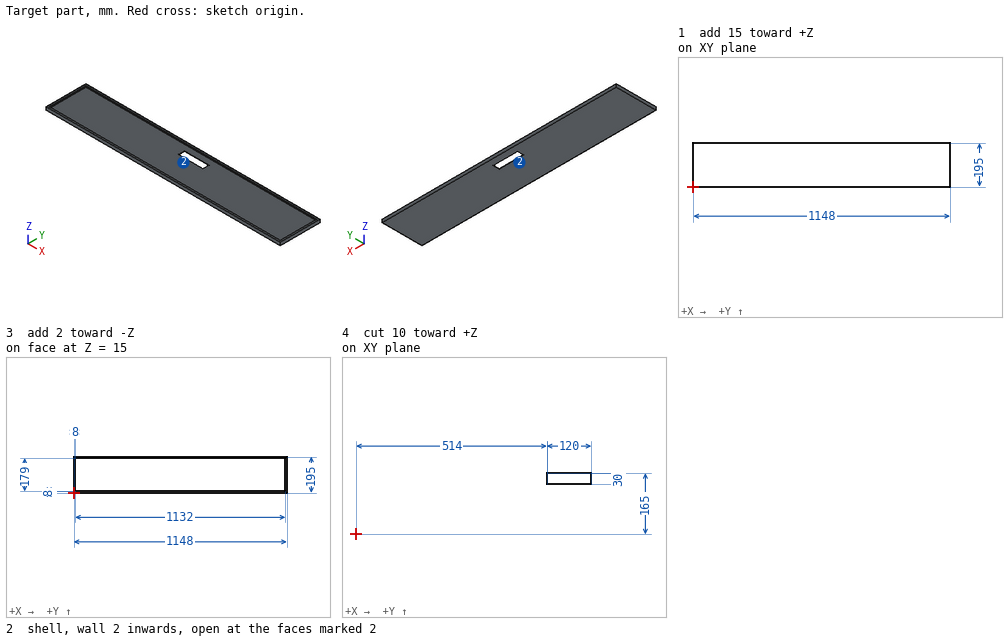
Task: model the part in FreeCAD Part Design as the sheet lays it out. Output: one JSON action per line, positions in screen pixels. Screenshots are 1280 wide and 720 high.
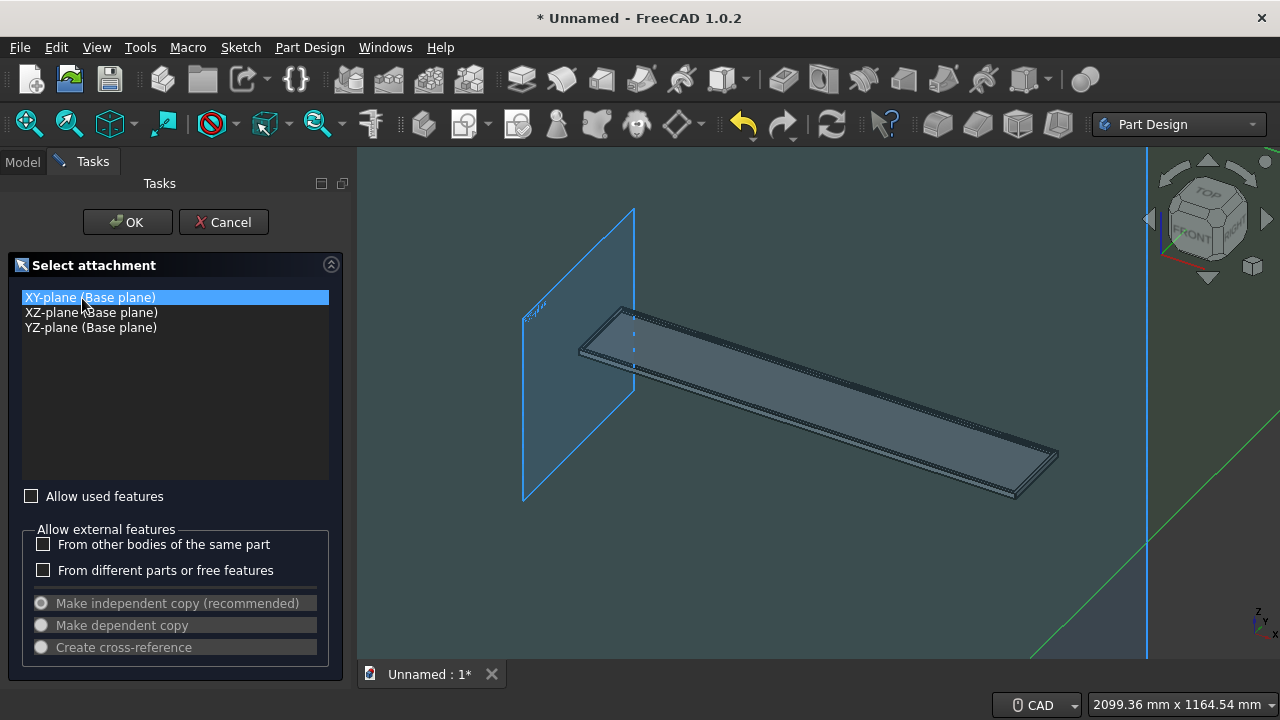
{"action": "left_click", "coordinate": [128, 222]}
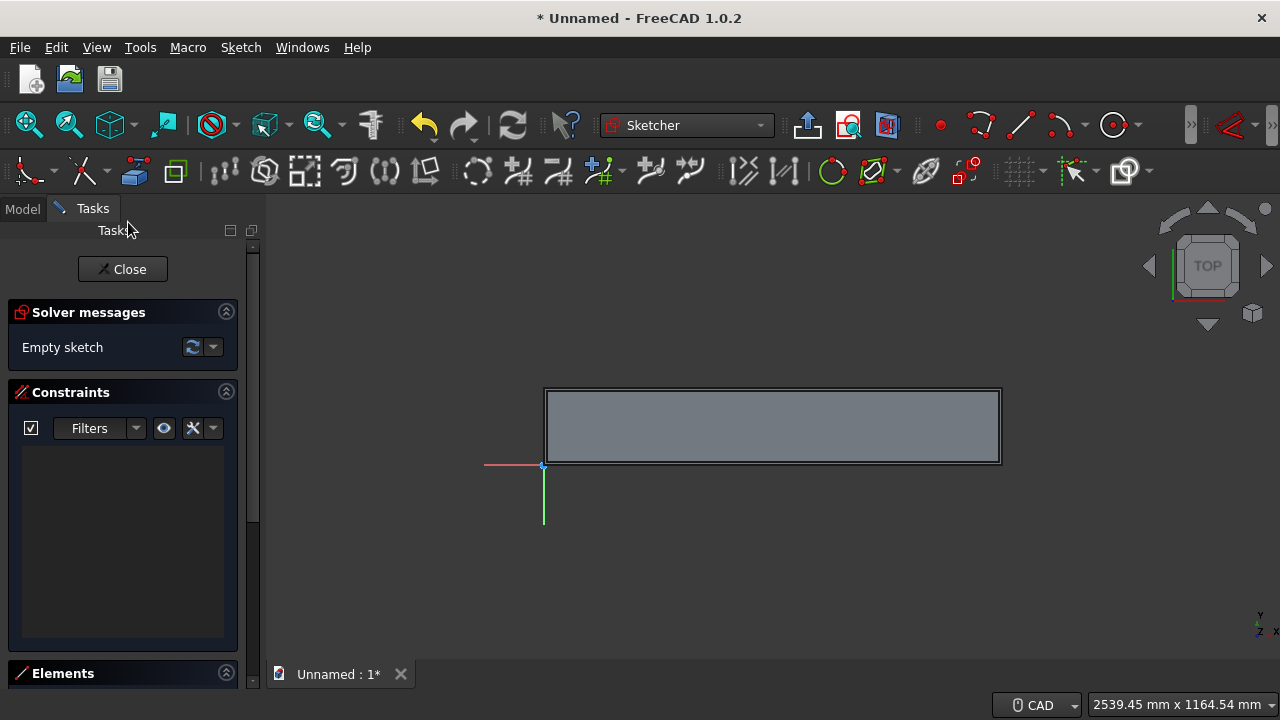
{"action": "key", "text": "q s"}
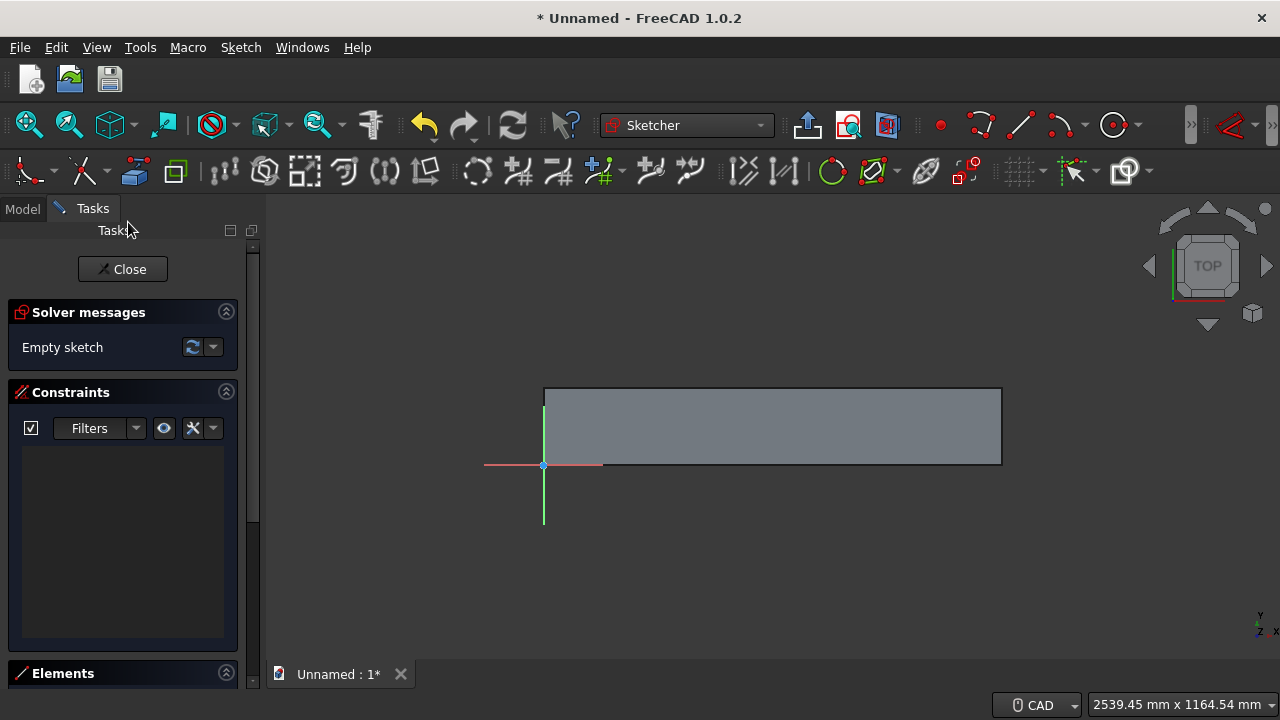
{"action": "scroll", "coordinate": [780, 403], "scroll_direction": "up", "scroll_amount": 12}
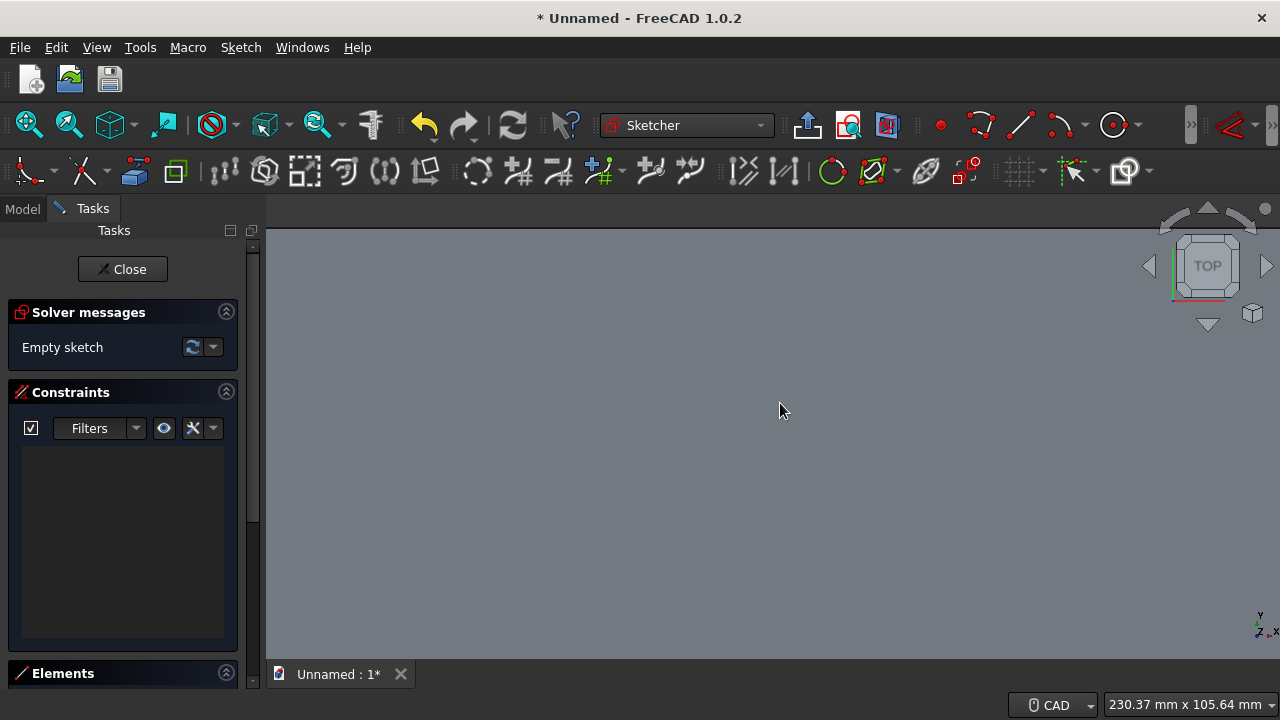
{"action": "key", "text": "g r"}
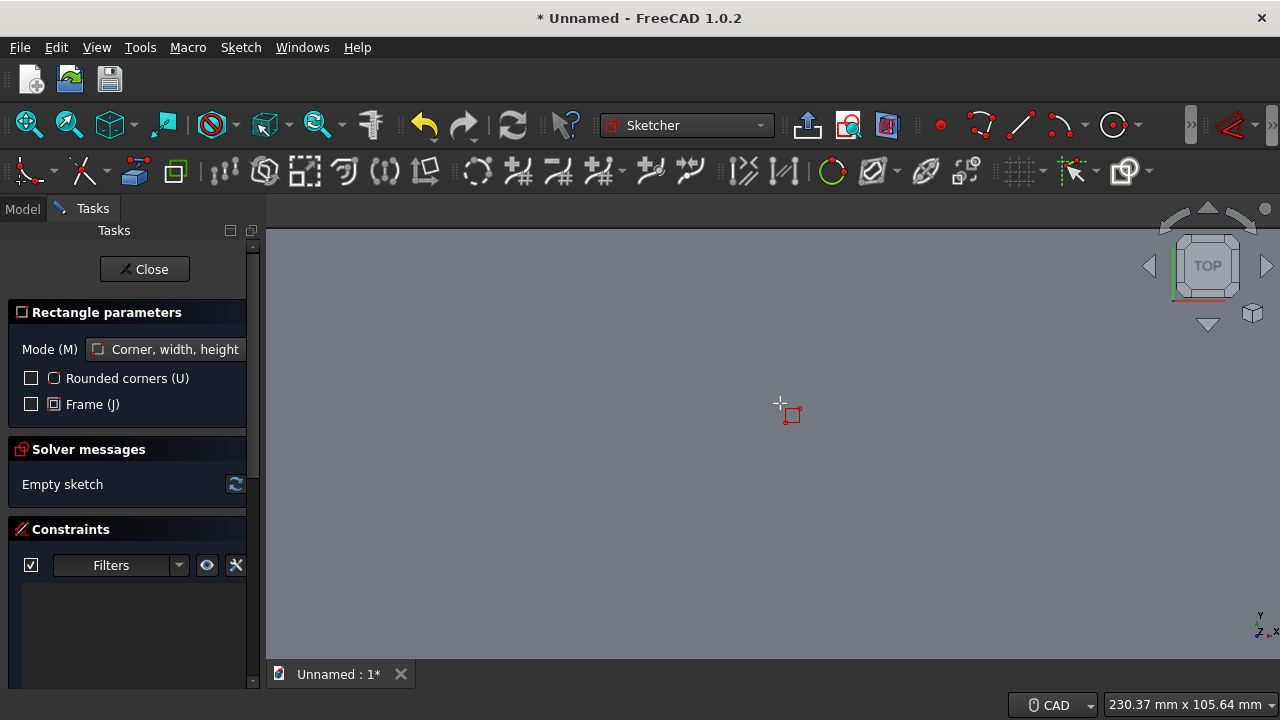
{"action": "left_click", "coordinate": [434, 360]}
{"action": "mouse_move", "coordinate": [962, 492]}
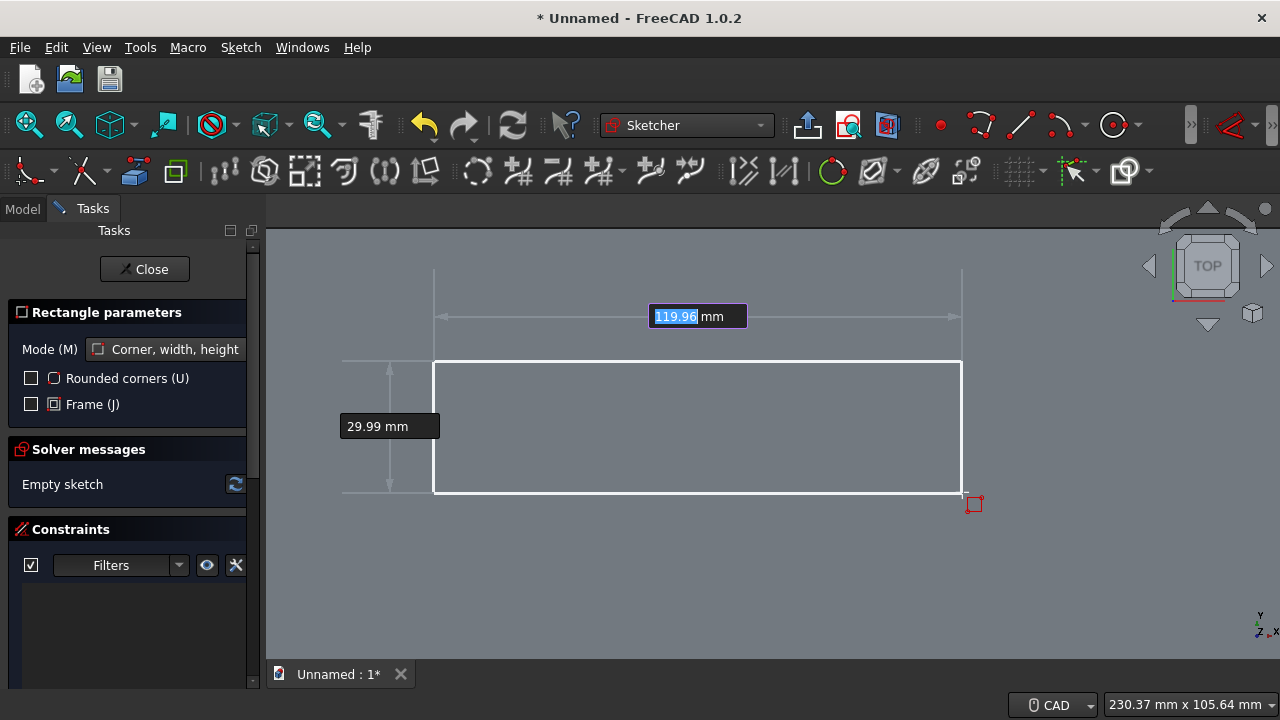
{"action": "type", "text": "120"}
{"action": "key", "text": "Tab"}
{"action": "type", "text": "30"}
{"action": "key", "text": "Return"}
{"action": "key", "text": "Escape"}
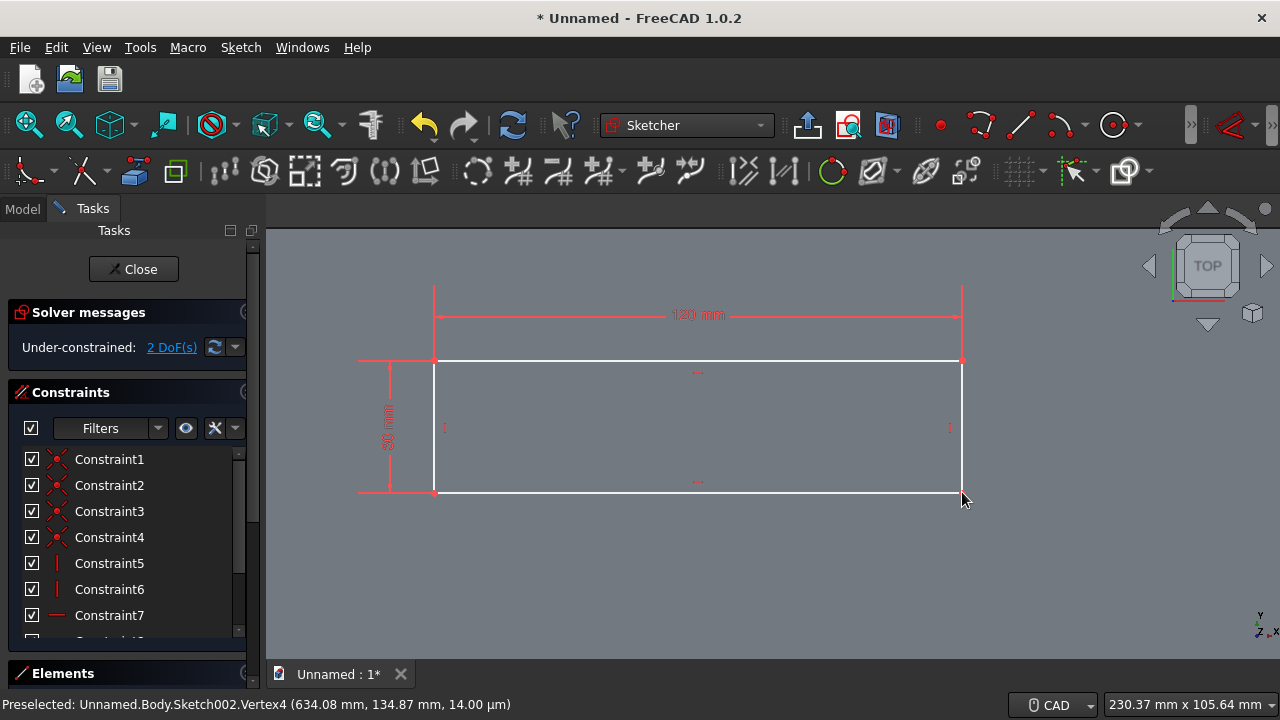
{"action": "key", "text": "d"}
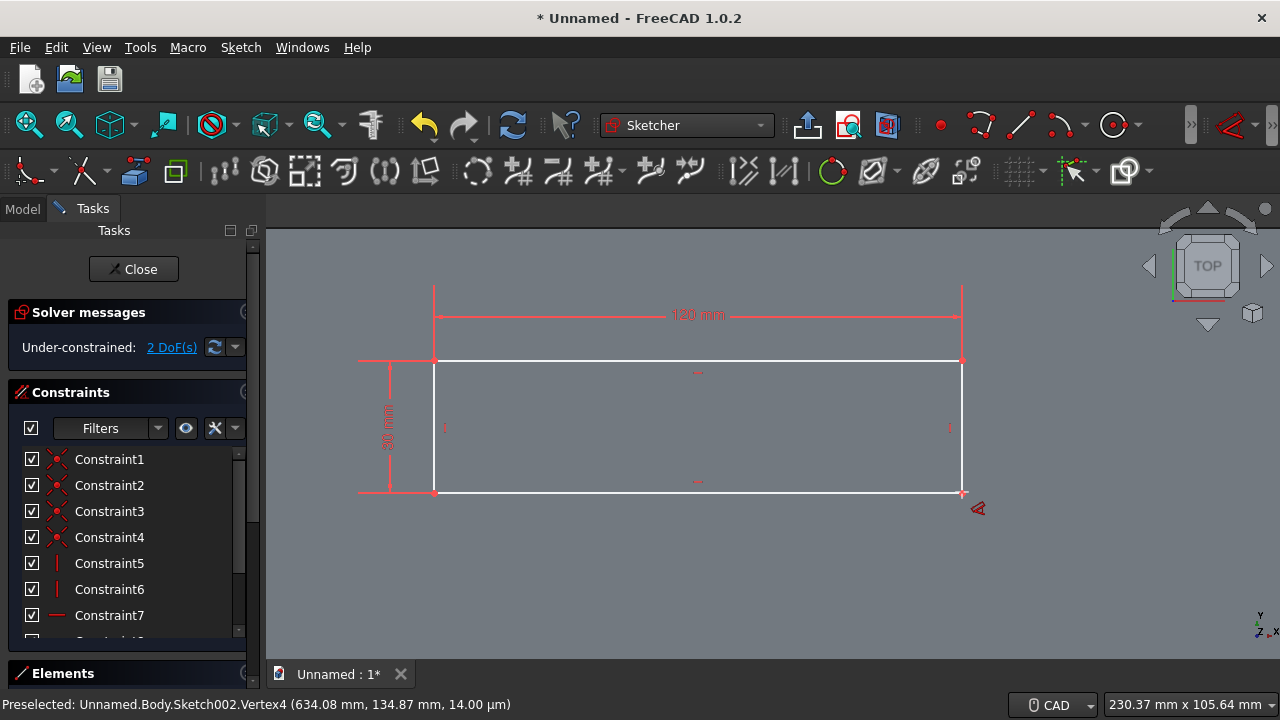
{"action": "left_click", "coordinate": [434, 361]}
{"action": "left_click", "coordinate": [364, 327]}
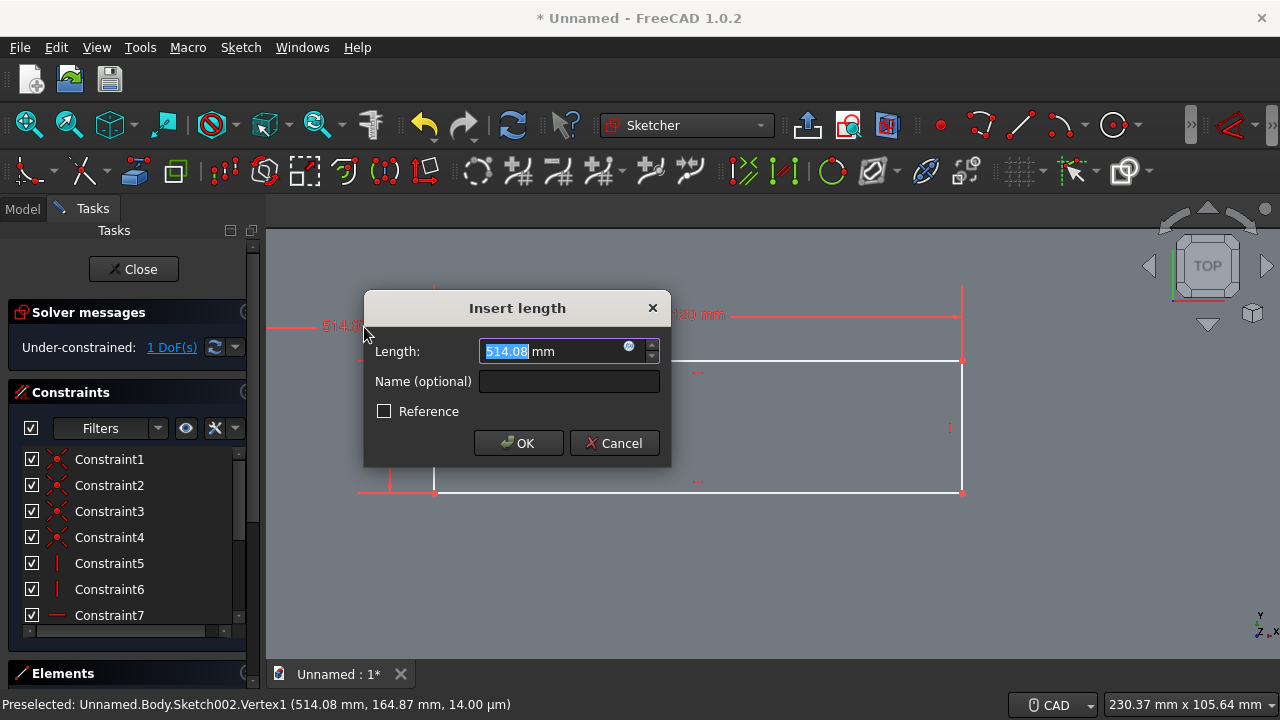
{"action": "type", "text": "514"}
{"action": "key", "text": "Return"}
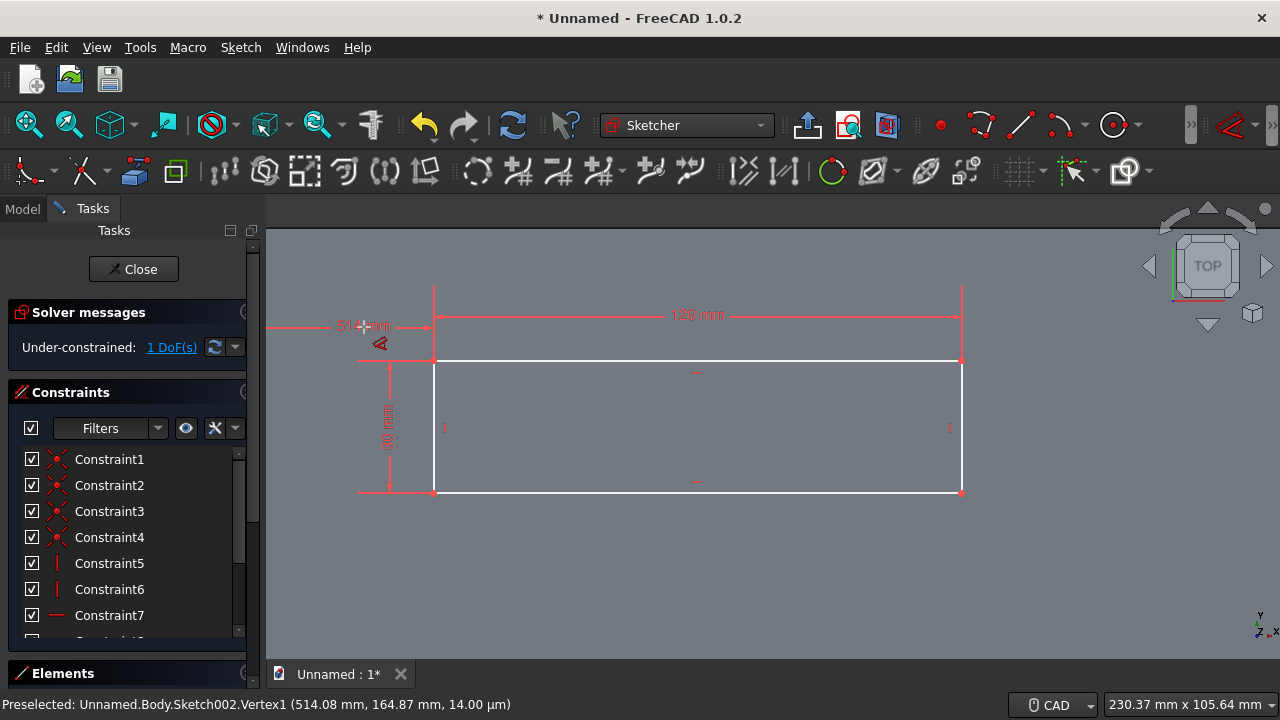
{"action": "left_click", "coordinate": [434, 361]}
{"action": "left_click", "coordinate": [468, 434]}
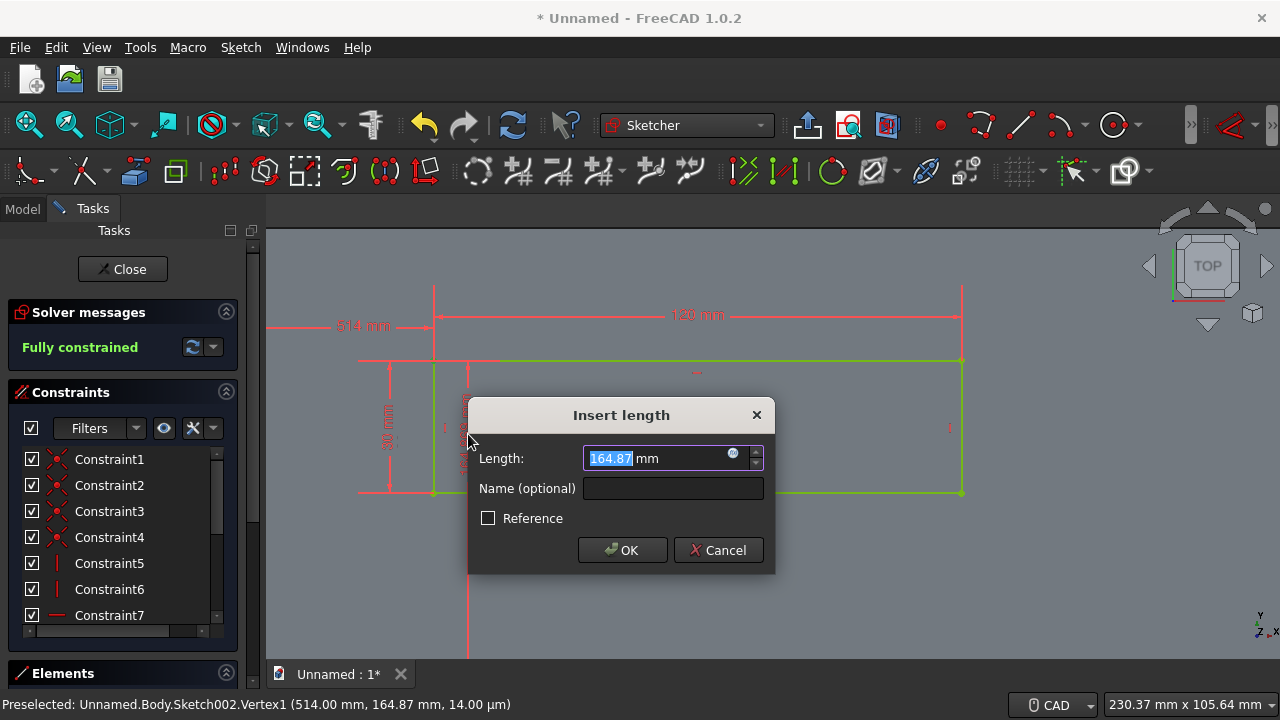
{"action": "type", "text": "165"}
{"action": "key", "text": "Return"}
{"action": "key", "text": "Escape"}